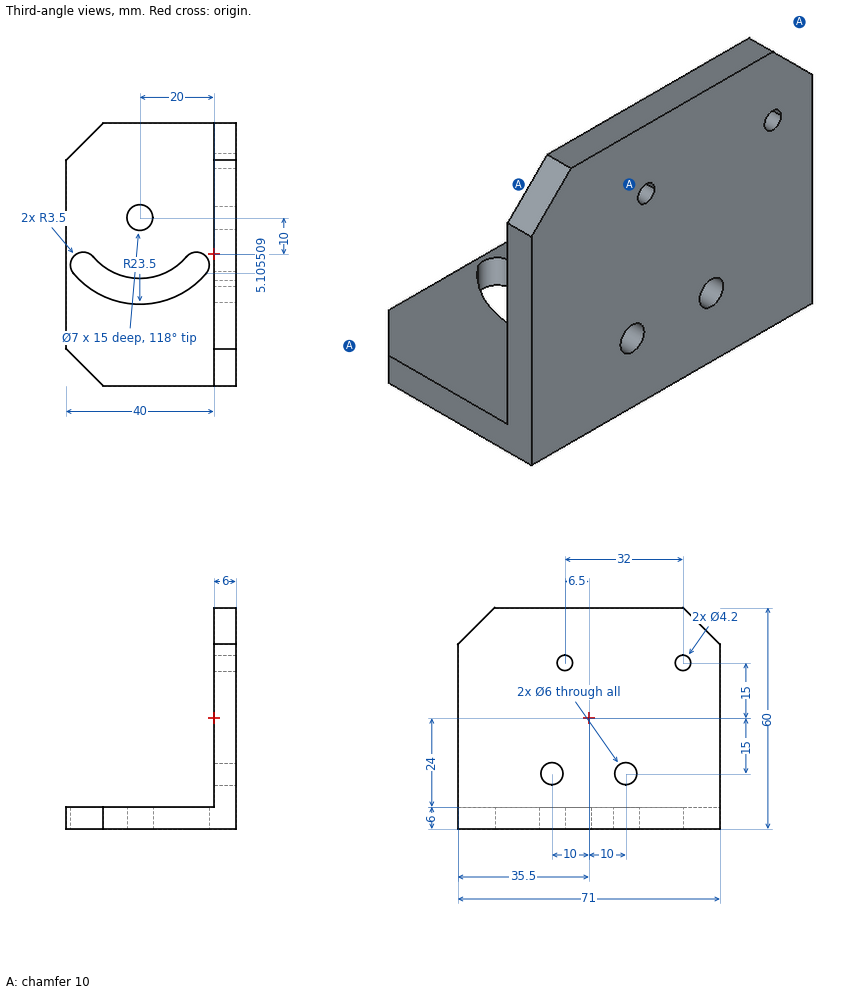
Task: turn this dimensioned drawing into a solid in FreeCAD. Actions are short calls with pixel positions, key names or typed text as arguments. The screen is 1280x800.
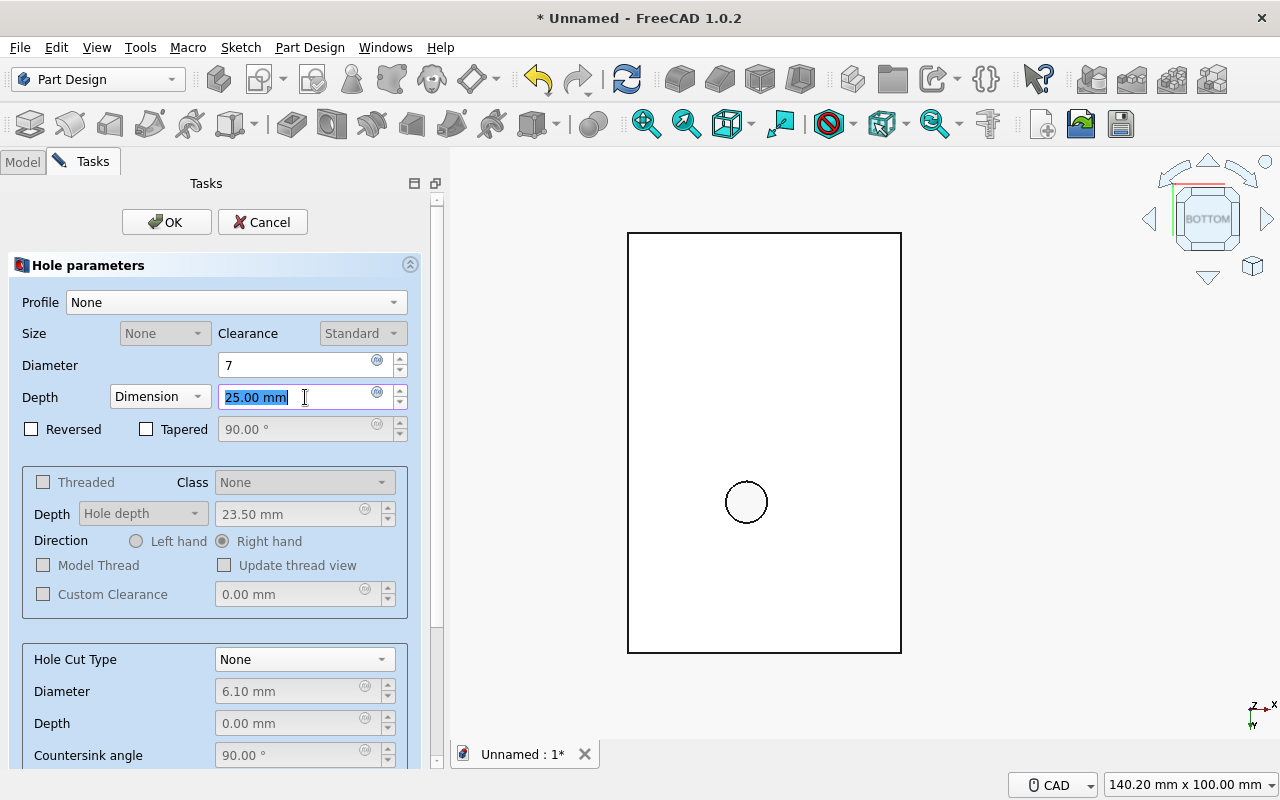
text(15)
key(Tab)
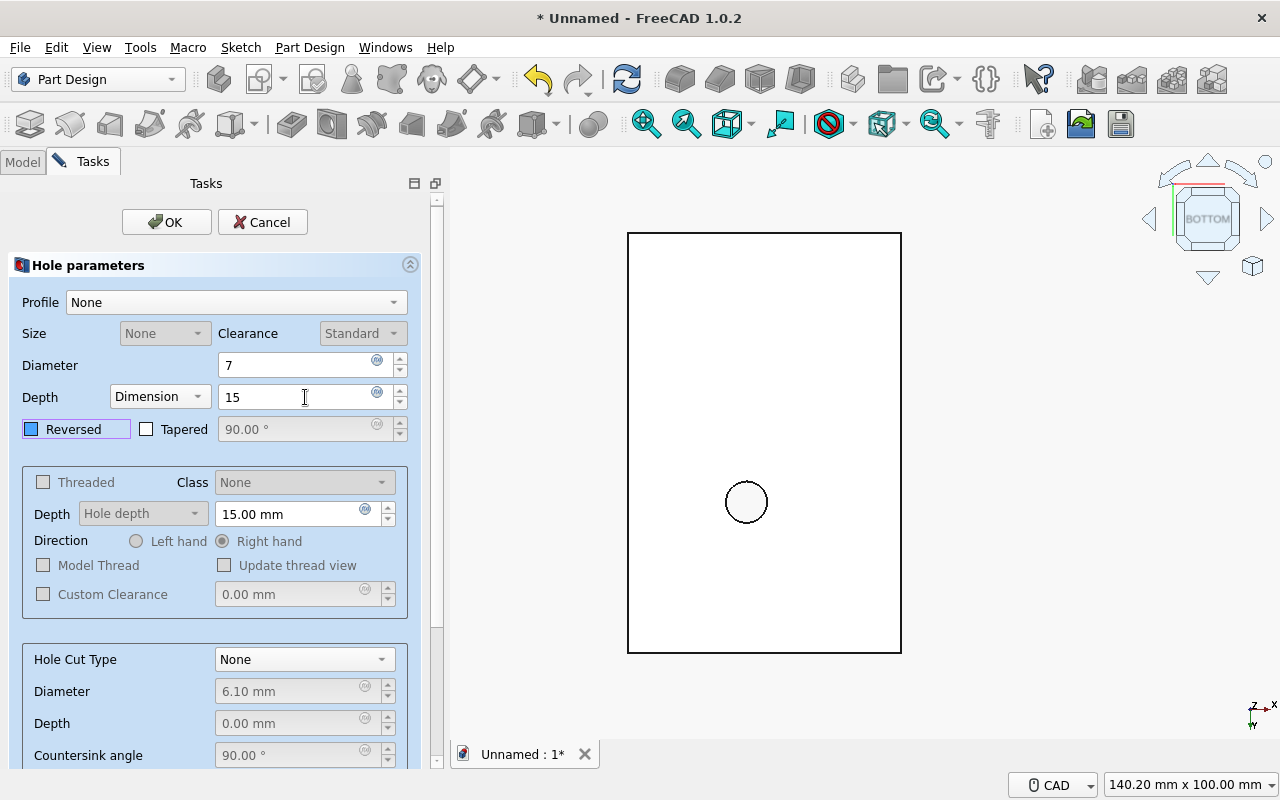
click(167, 222)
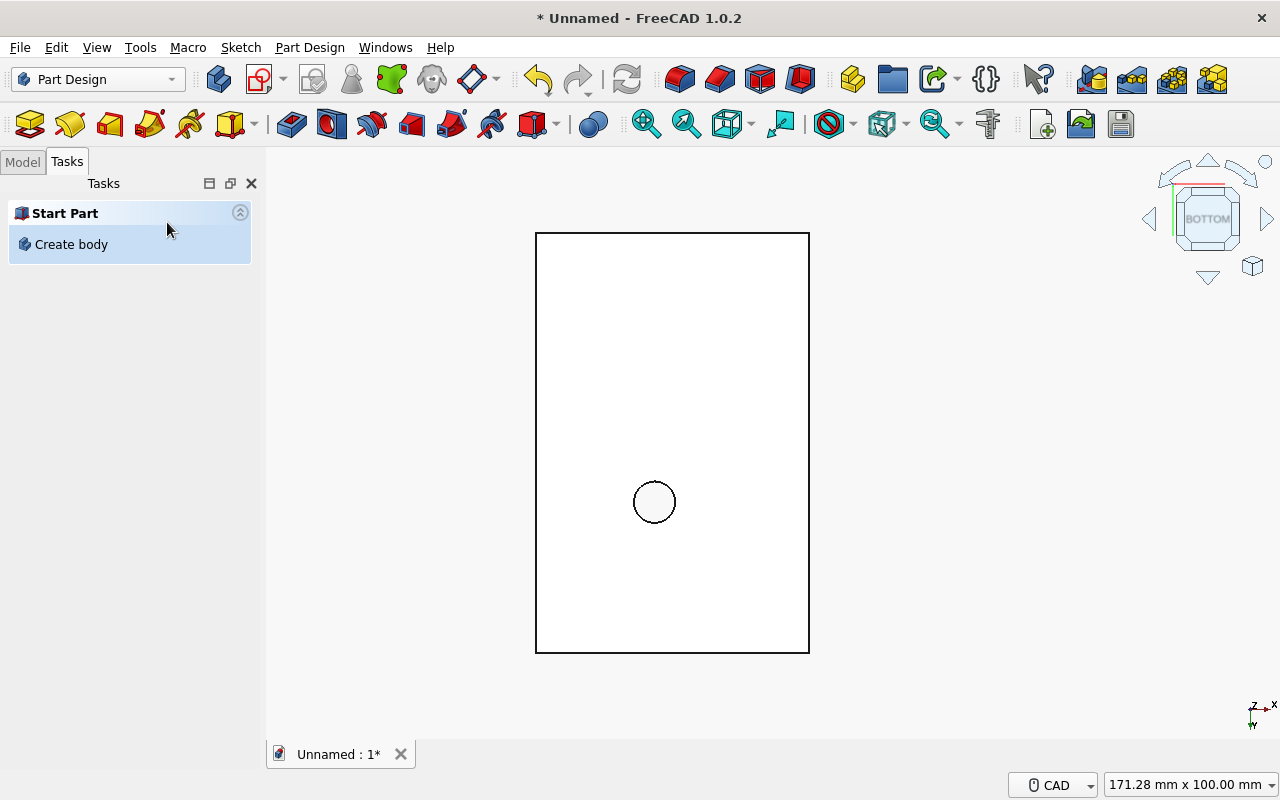
click(672, 382)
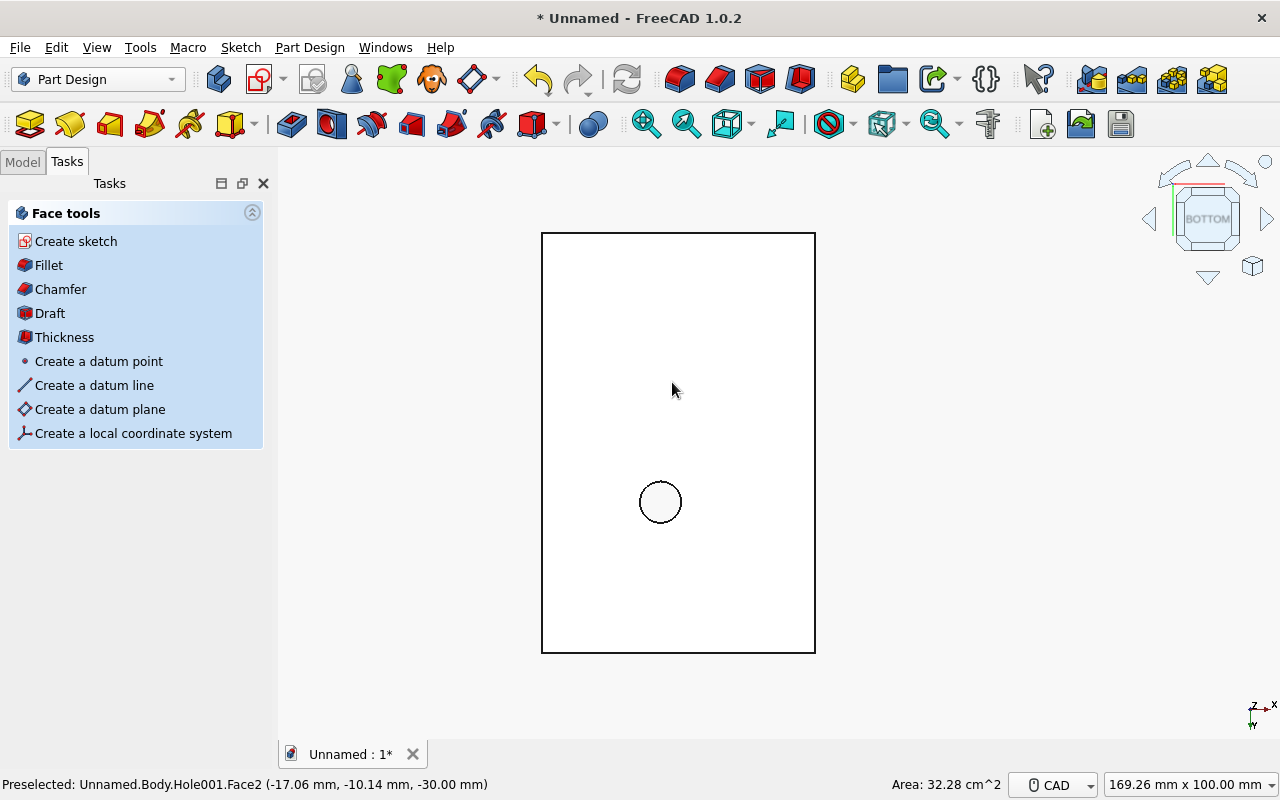
click(260, 80)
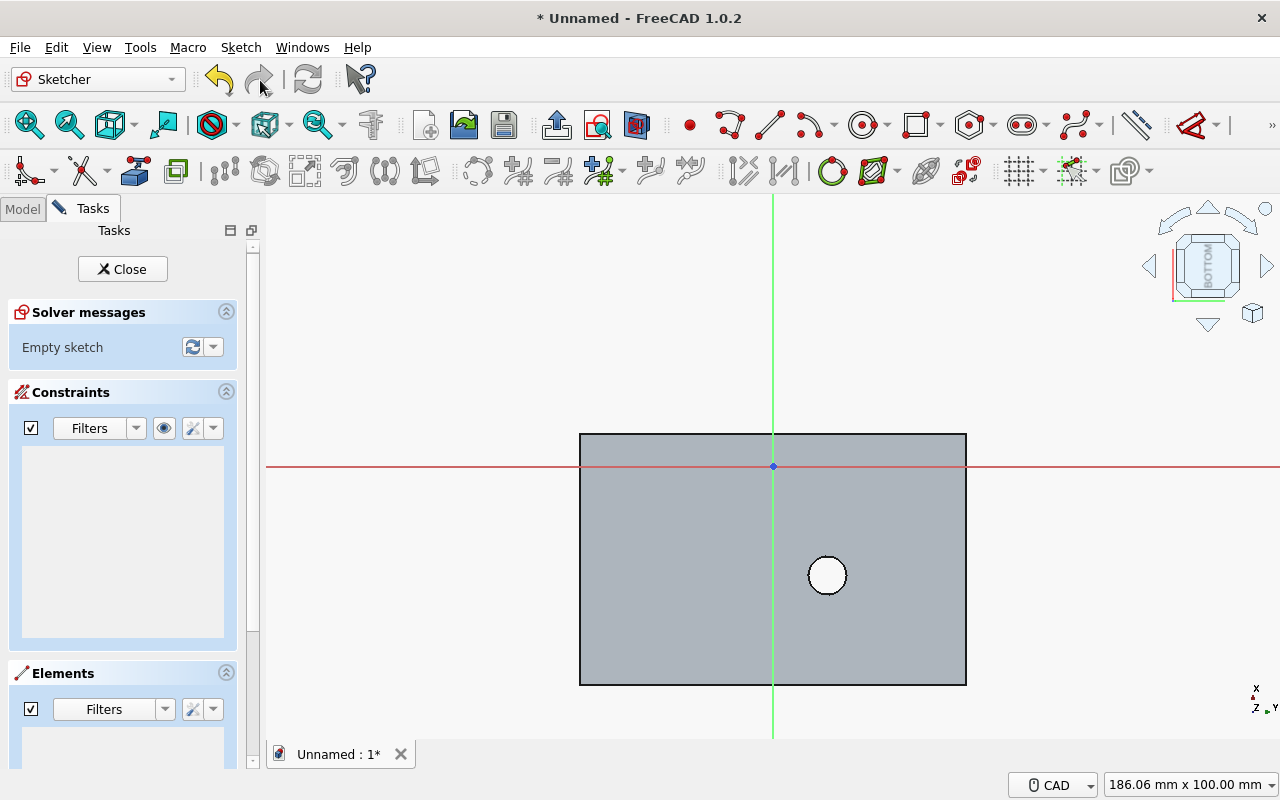
scroll(775, 696, up, 3)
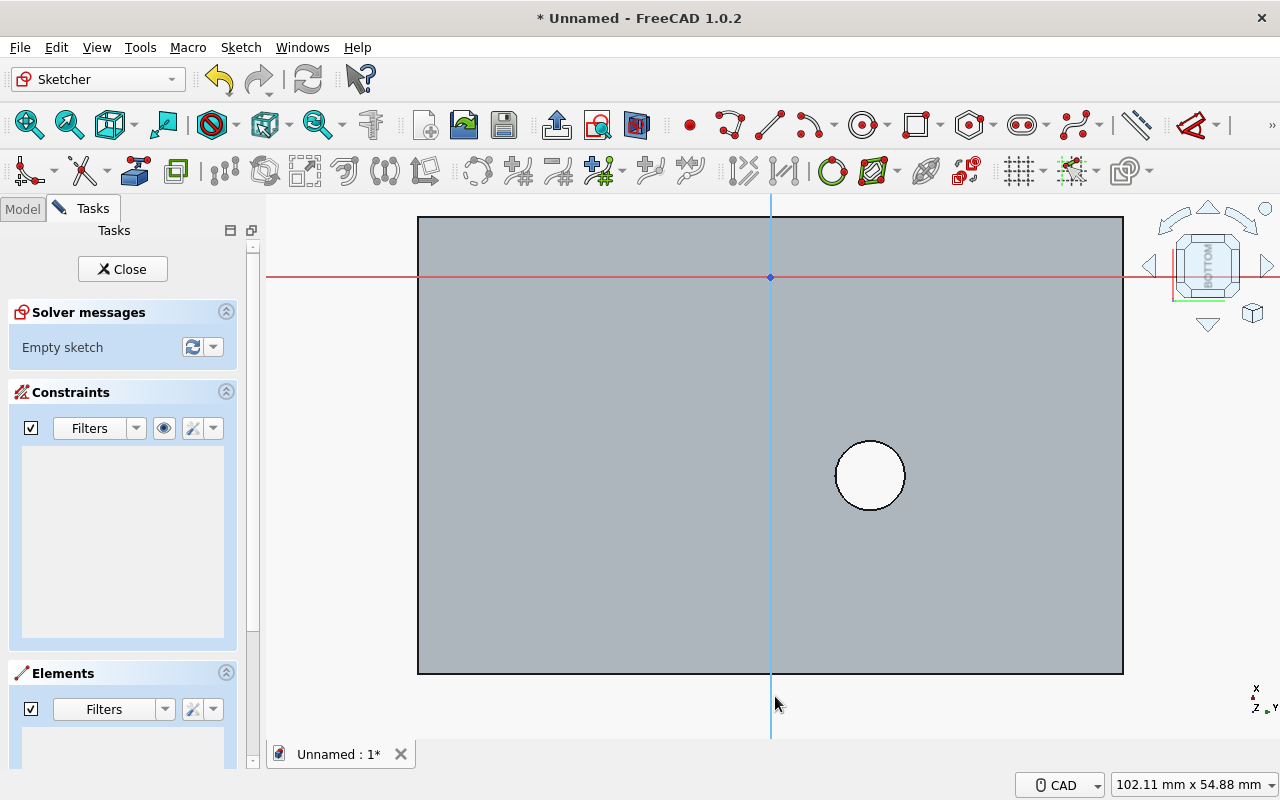
key(g)
key(3)
key(a)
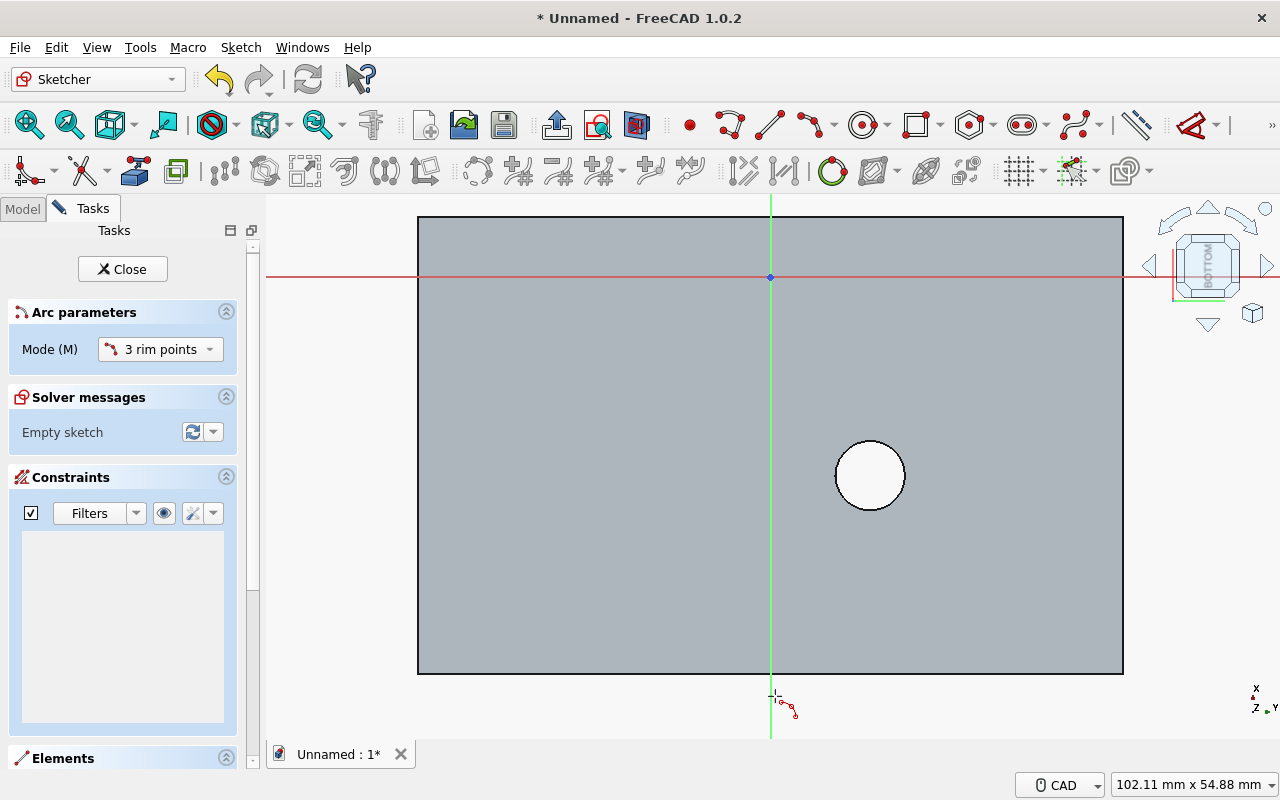
click(720, 297)
click(720, 654)
click(637, 476)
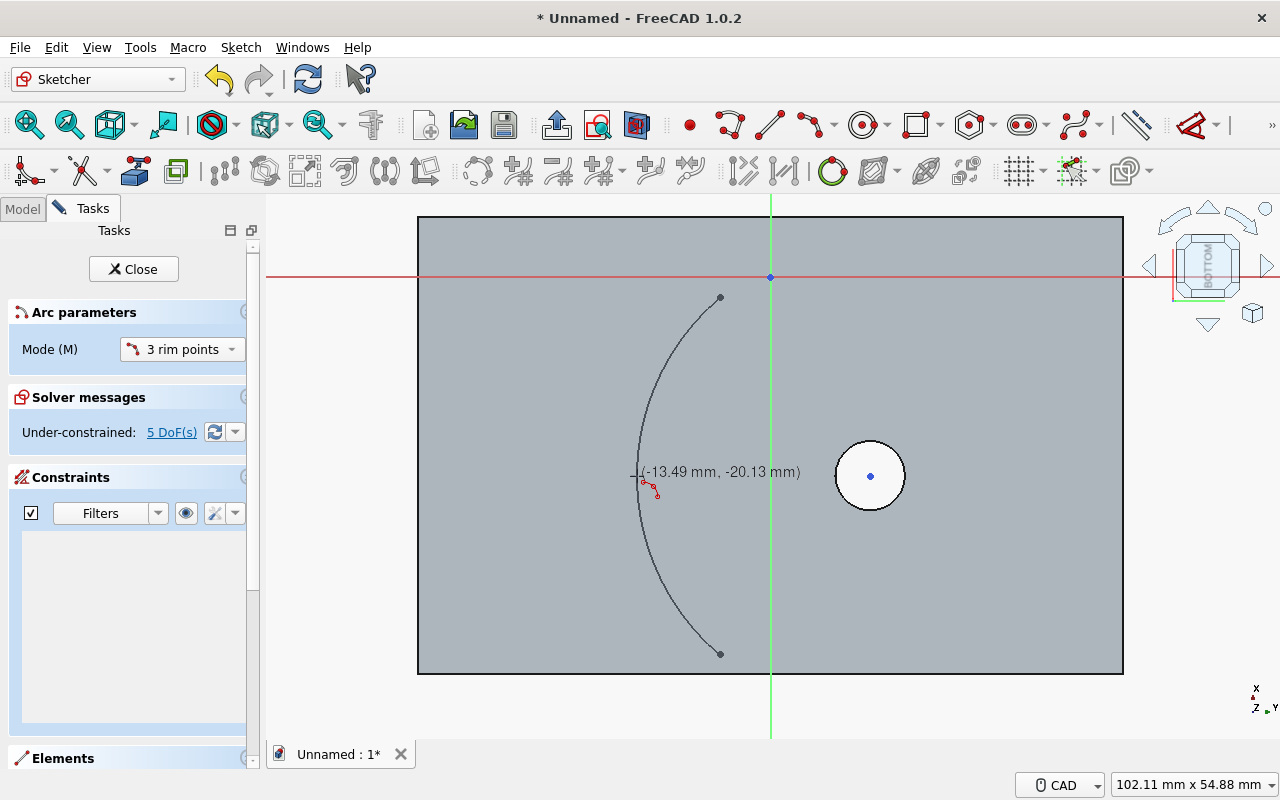
click(720, 655)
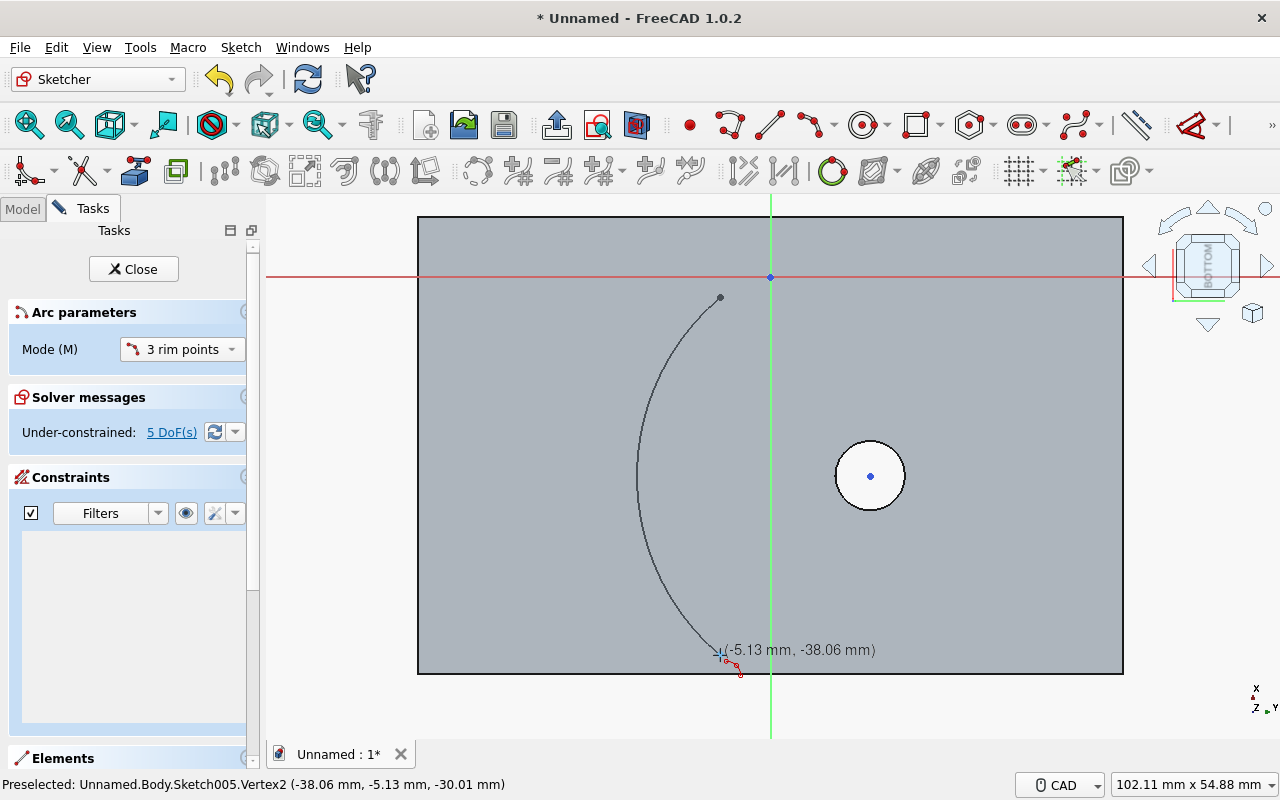
scroll(765, 601, up, 5)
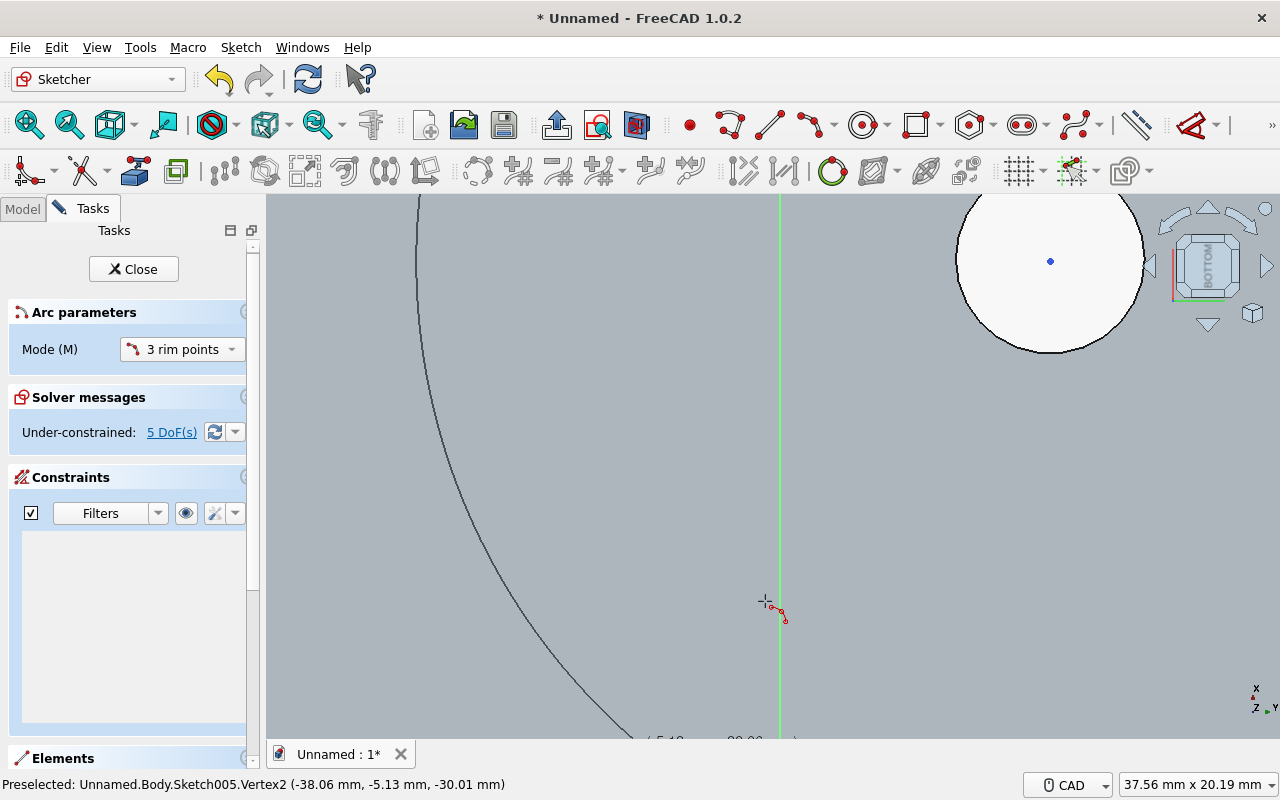
click(764, 600)